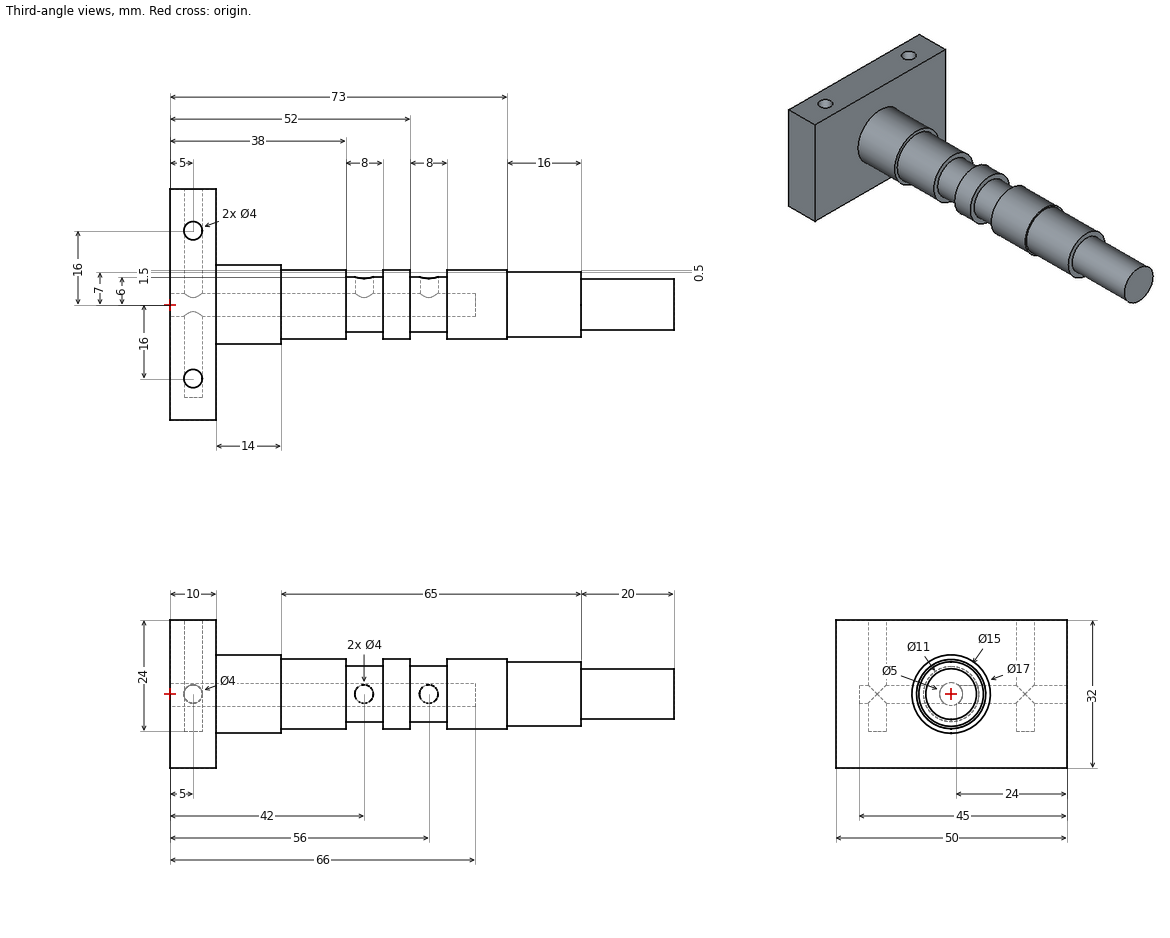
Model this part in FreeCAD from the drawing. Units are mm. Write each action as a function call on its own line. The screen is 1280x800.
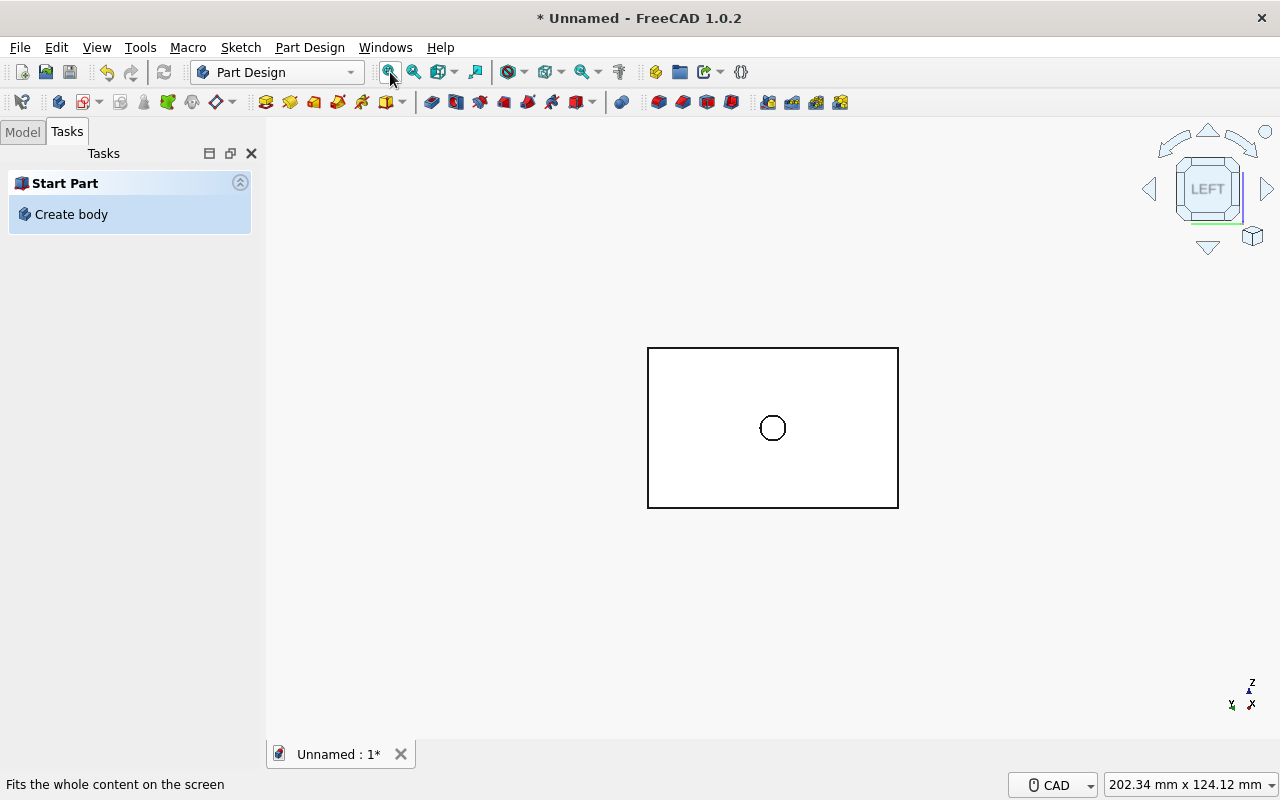
key(4)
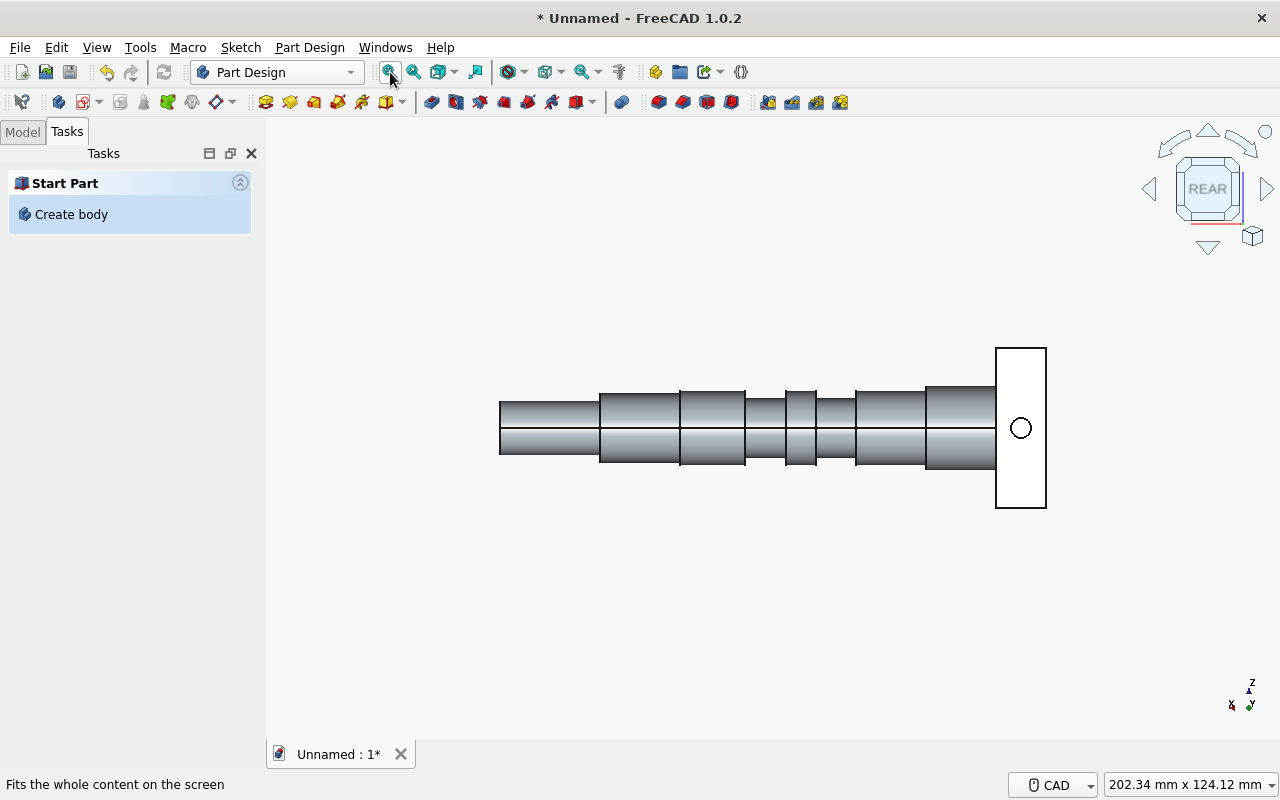
click(1021, 381)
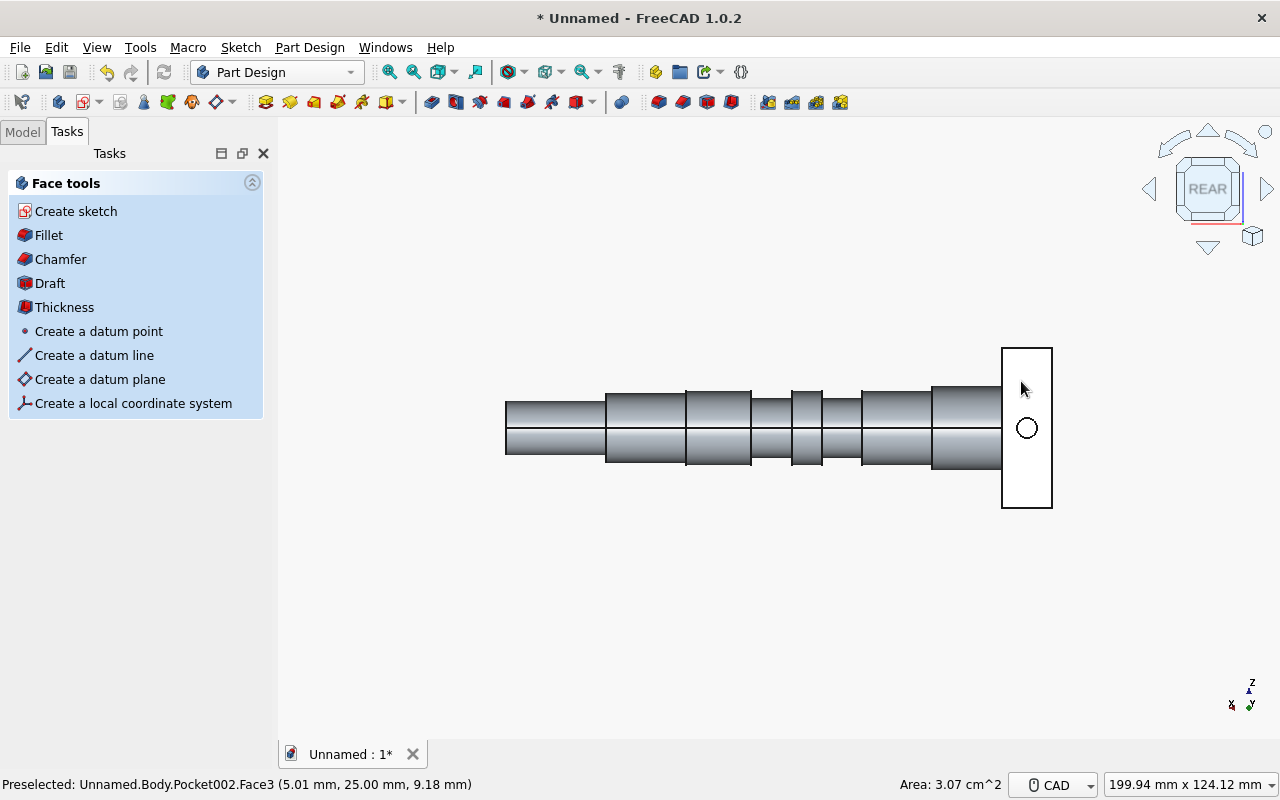
click(84, 102)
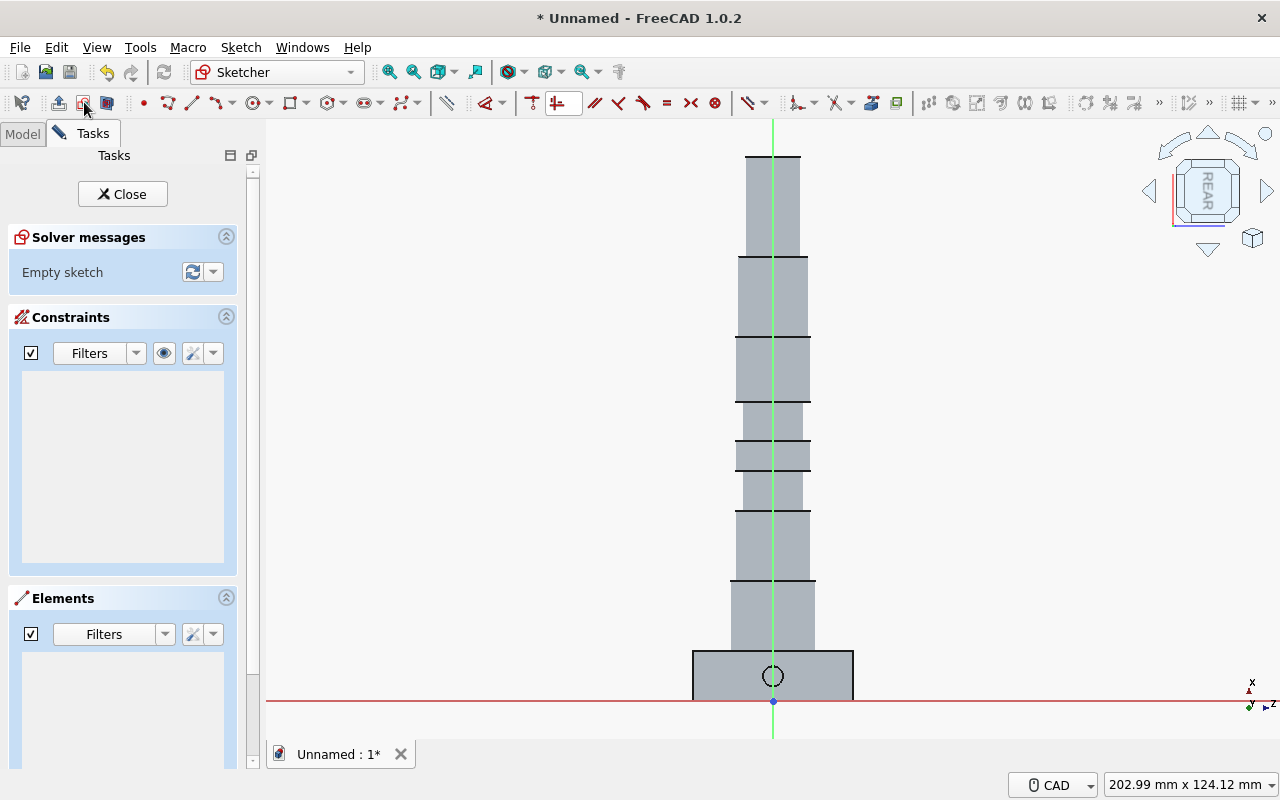
scroll(795, 465, up, 7)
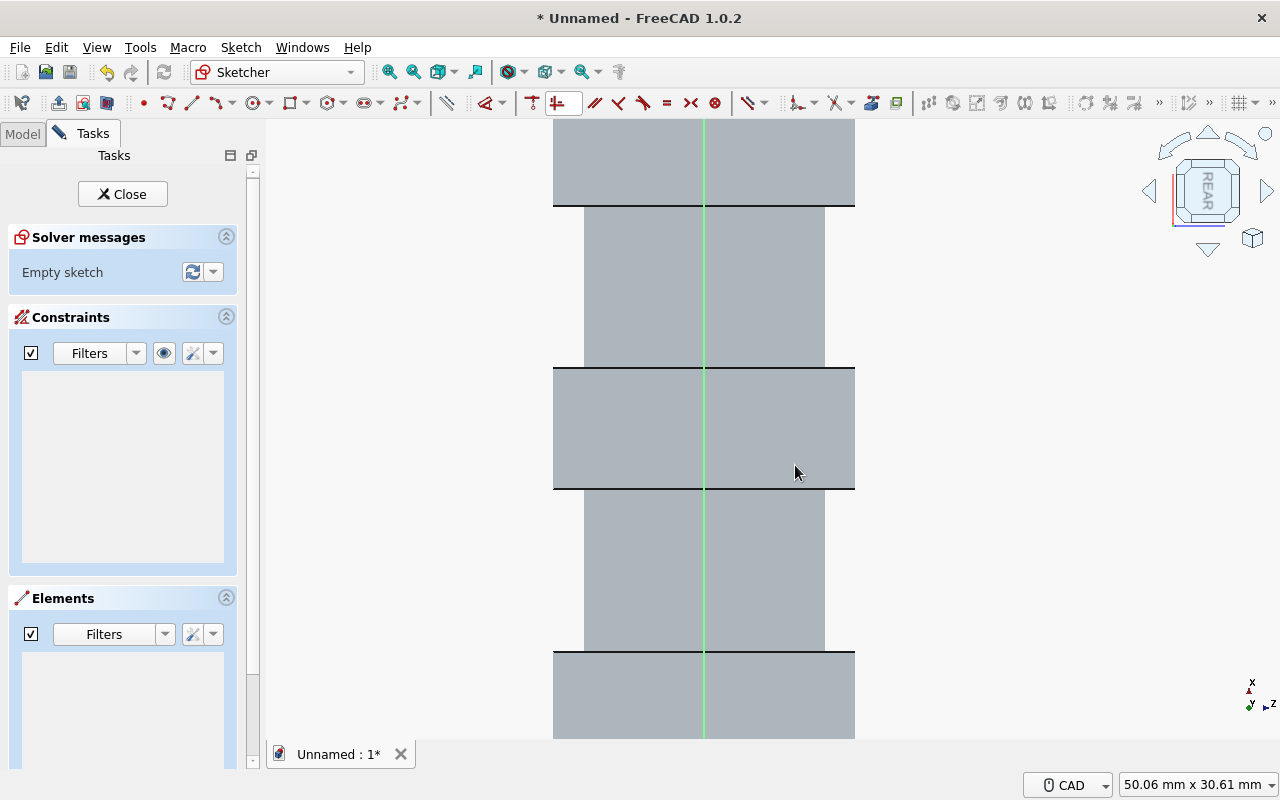
click(254, 104)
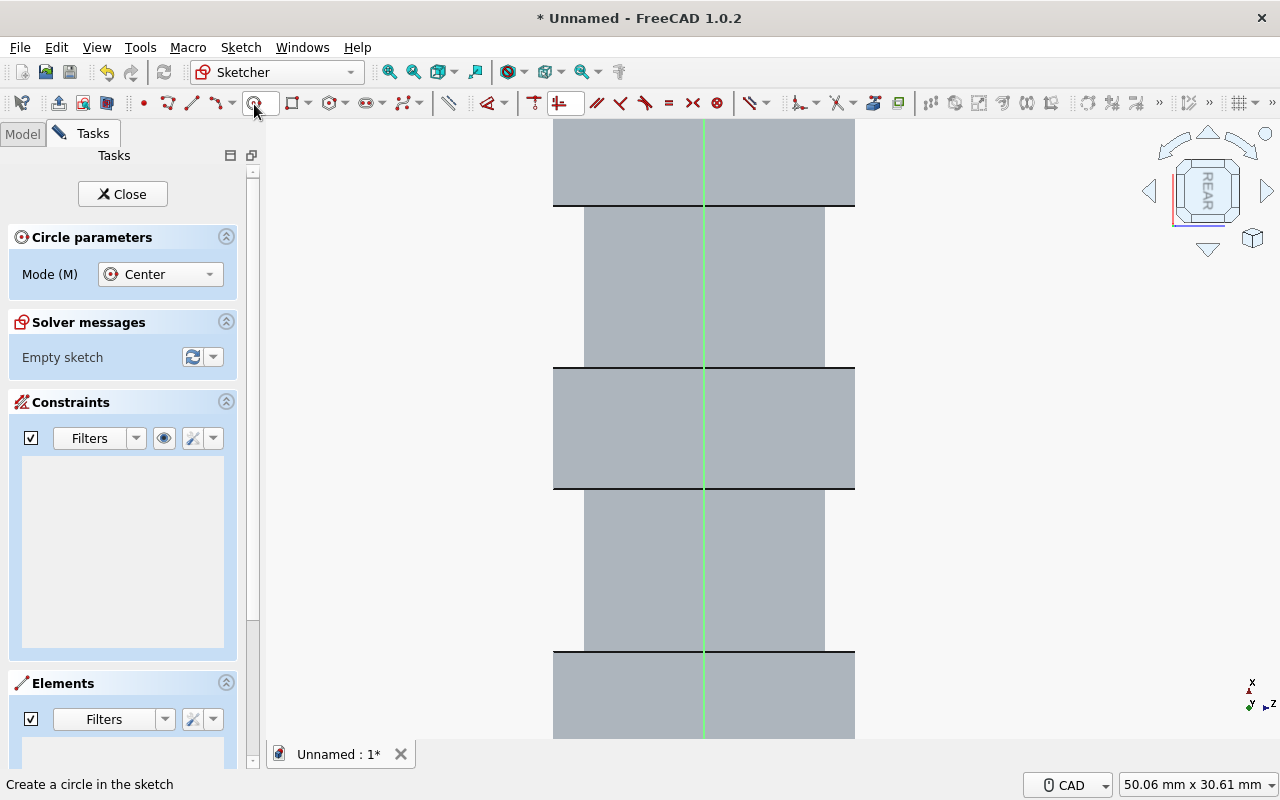
click(704, 571)
move(733, 542)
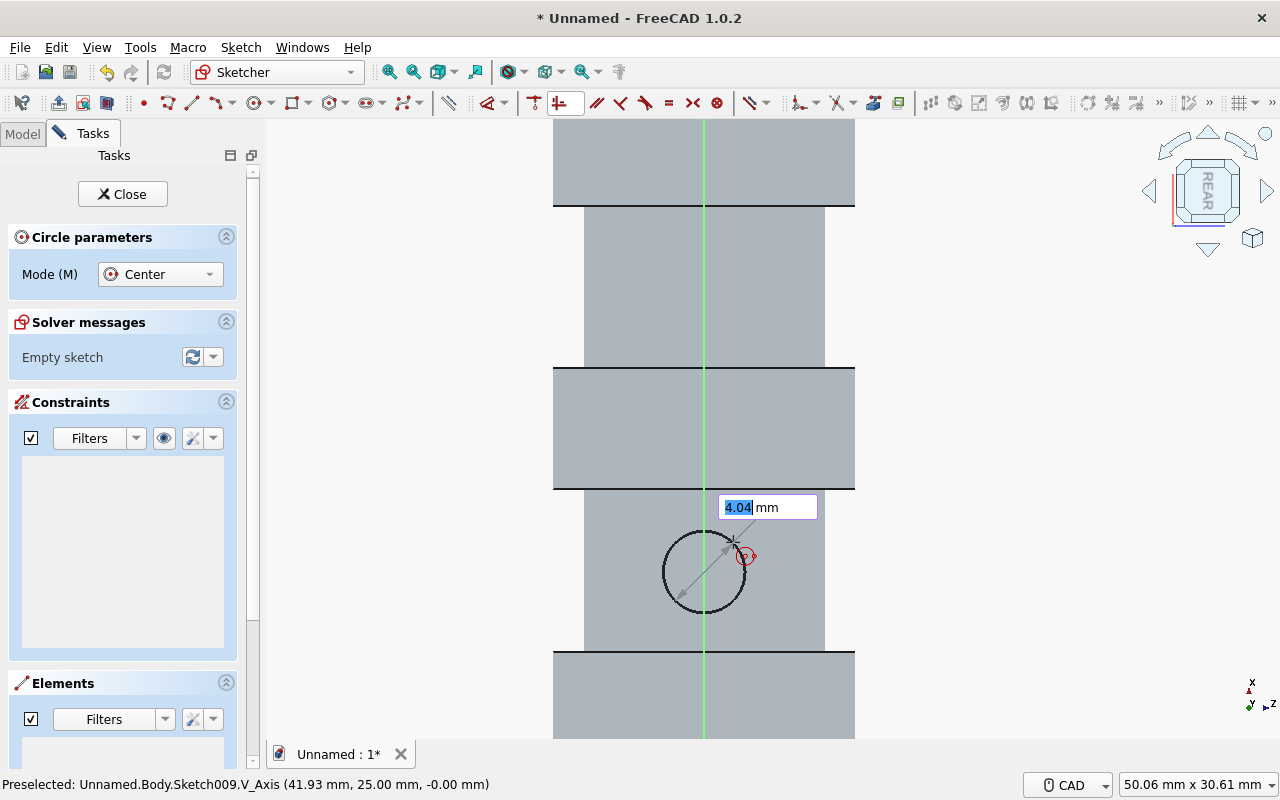
text(4)
key(Return)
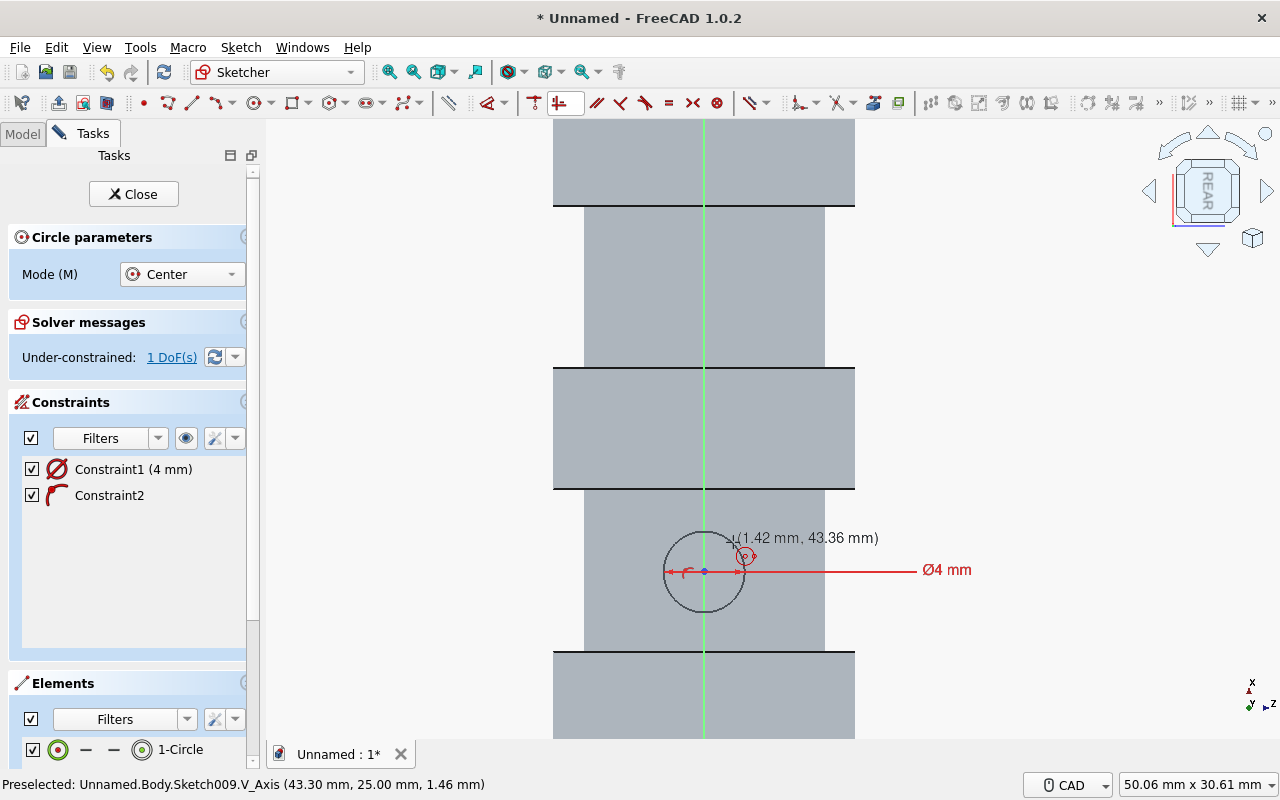
click(704, 287)
move(733, 258)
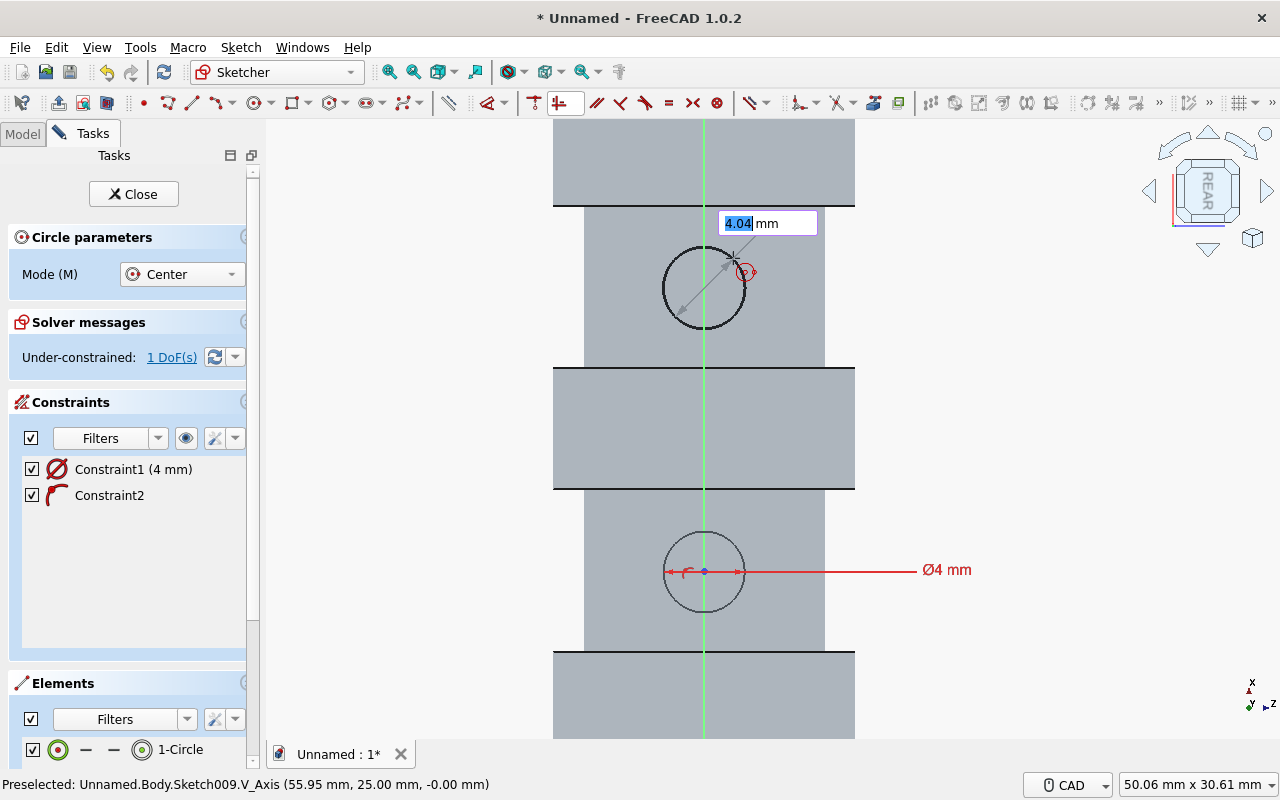
text(4)
key(Return)
key(Escape)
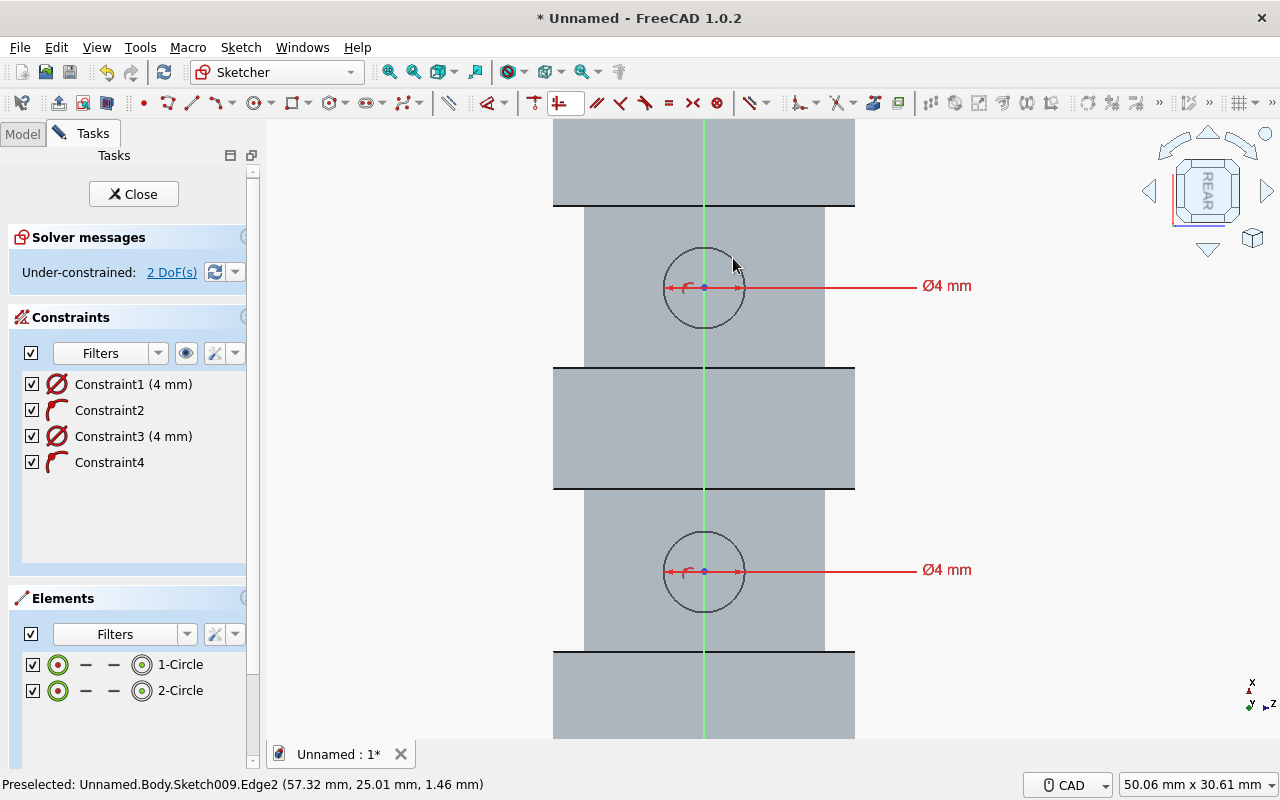
click(488, 104)